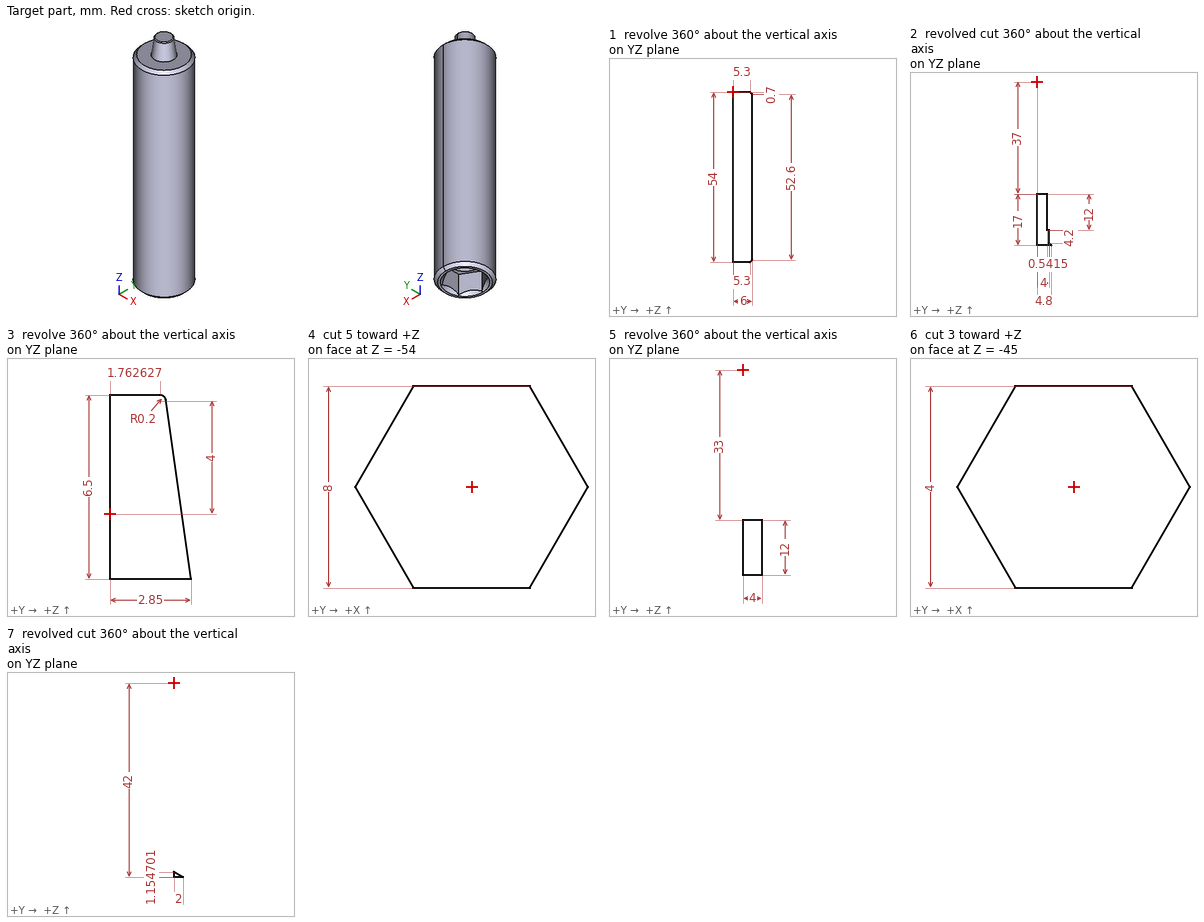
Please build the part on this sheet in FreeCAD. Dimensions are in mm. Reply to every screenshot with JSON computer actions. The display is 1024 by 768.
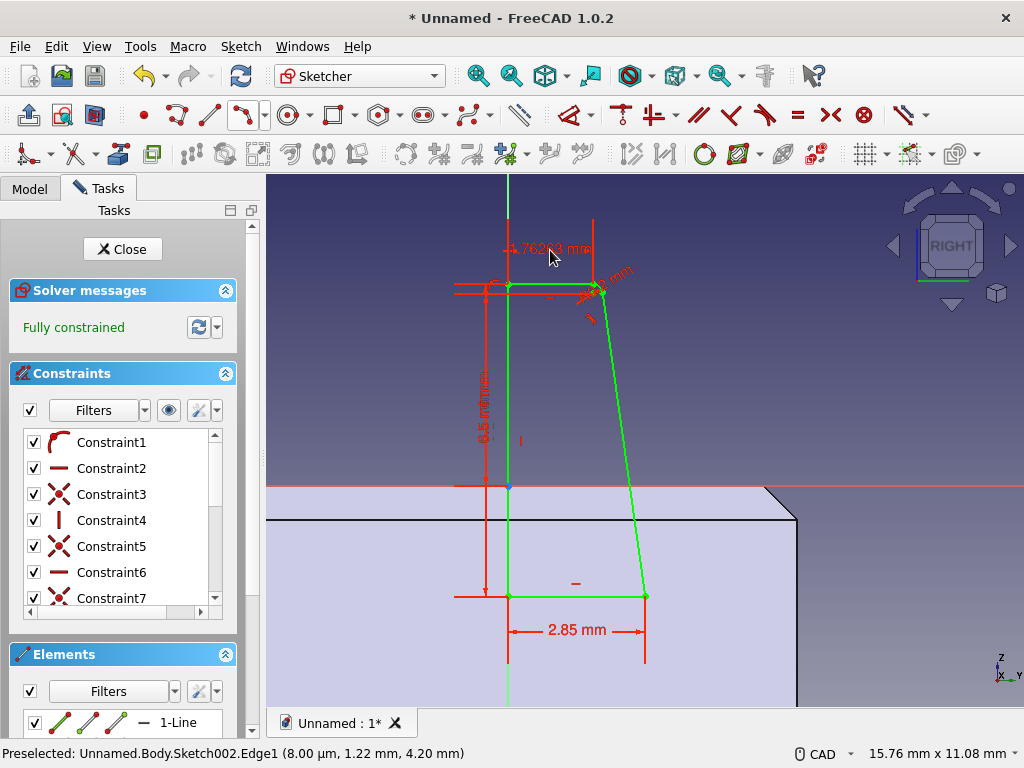
{"action": "left_click", "coordinate": [123, 249]}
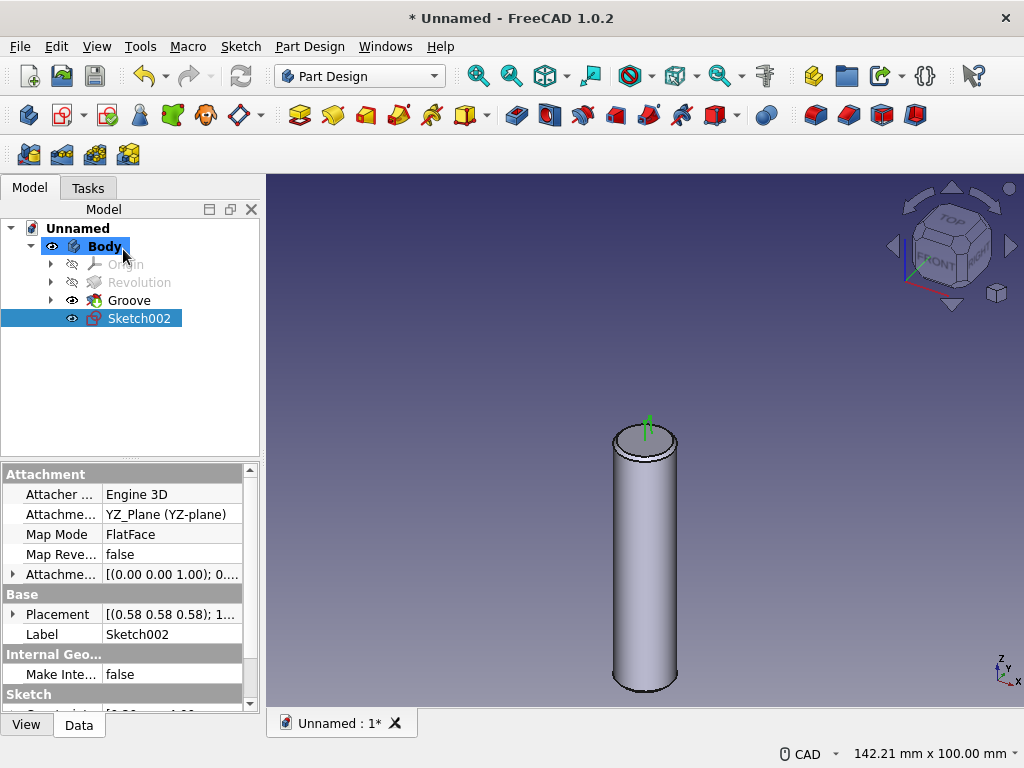
{"action": "left_click", "coordinate": [333, 116]}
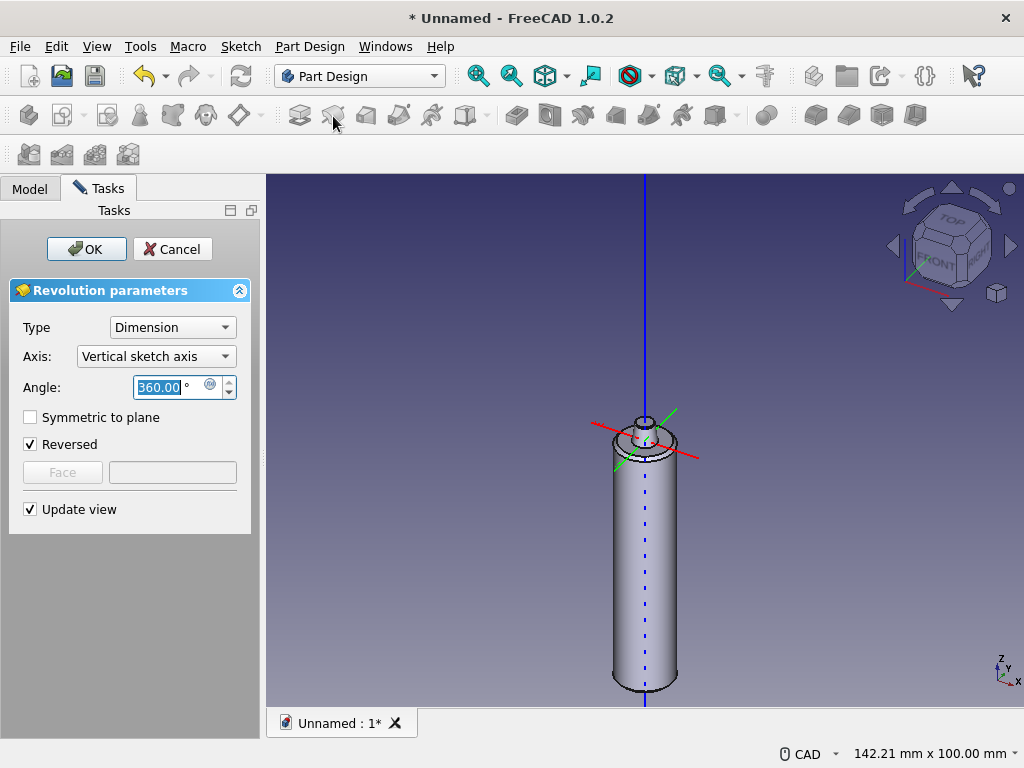
{"action": "left_click", "coordinate": [87, 249]}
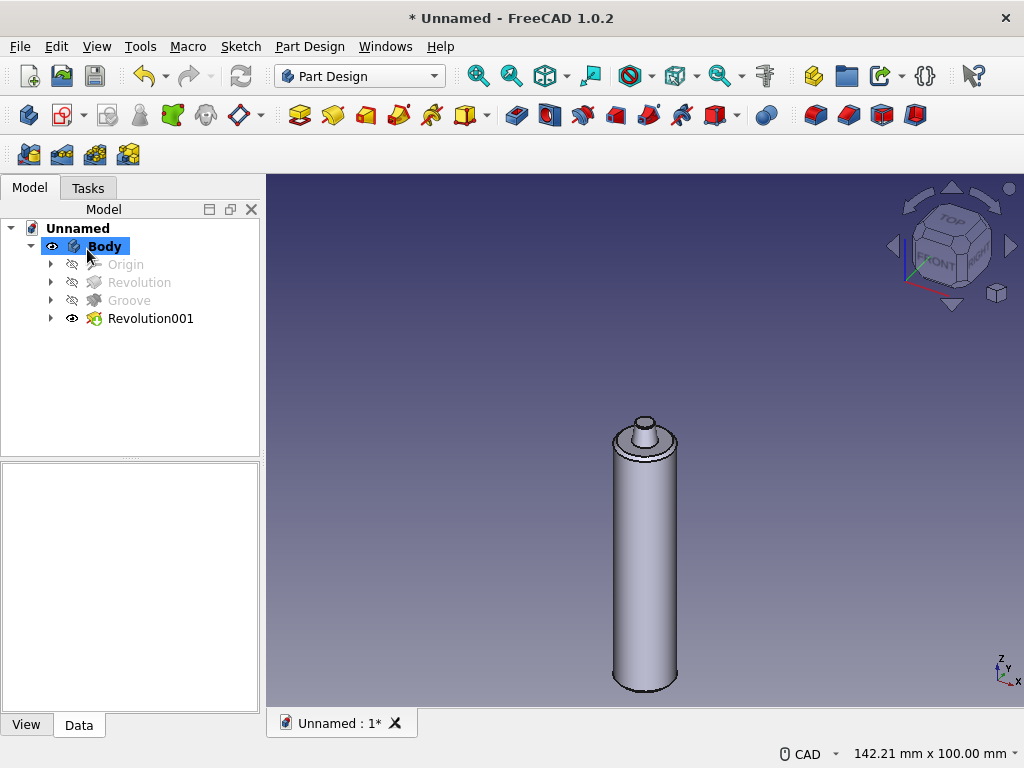
{"action": "key", "text": "5"}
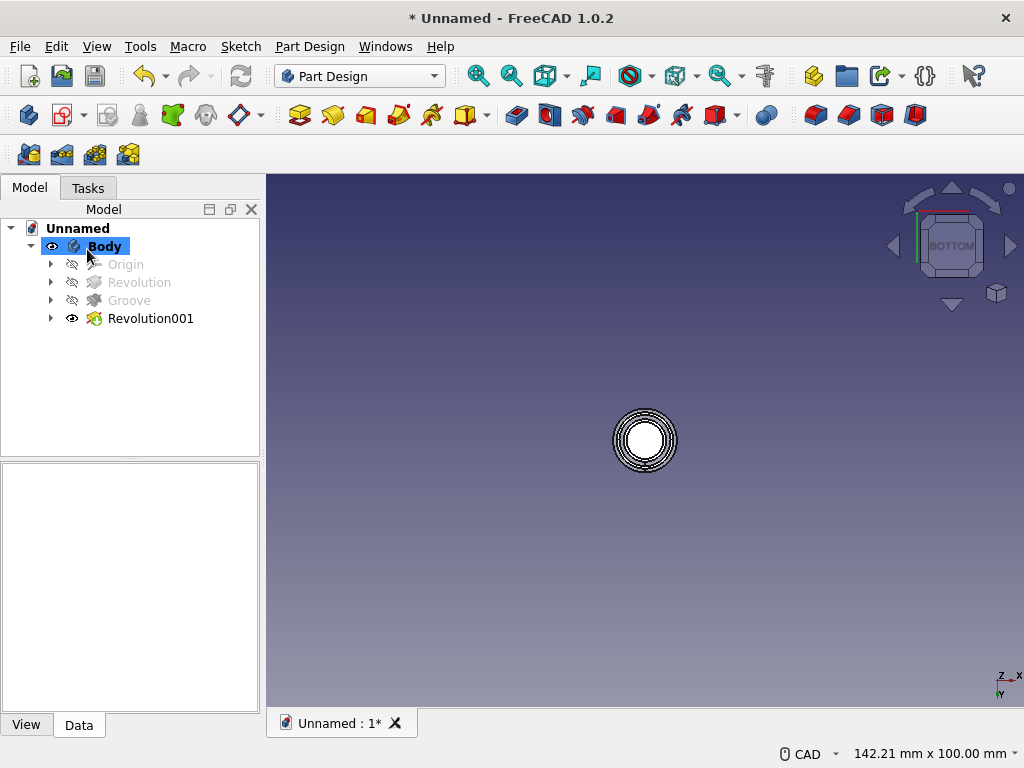
{"action": "left_click", "coordinate": [479, 76]}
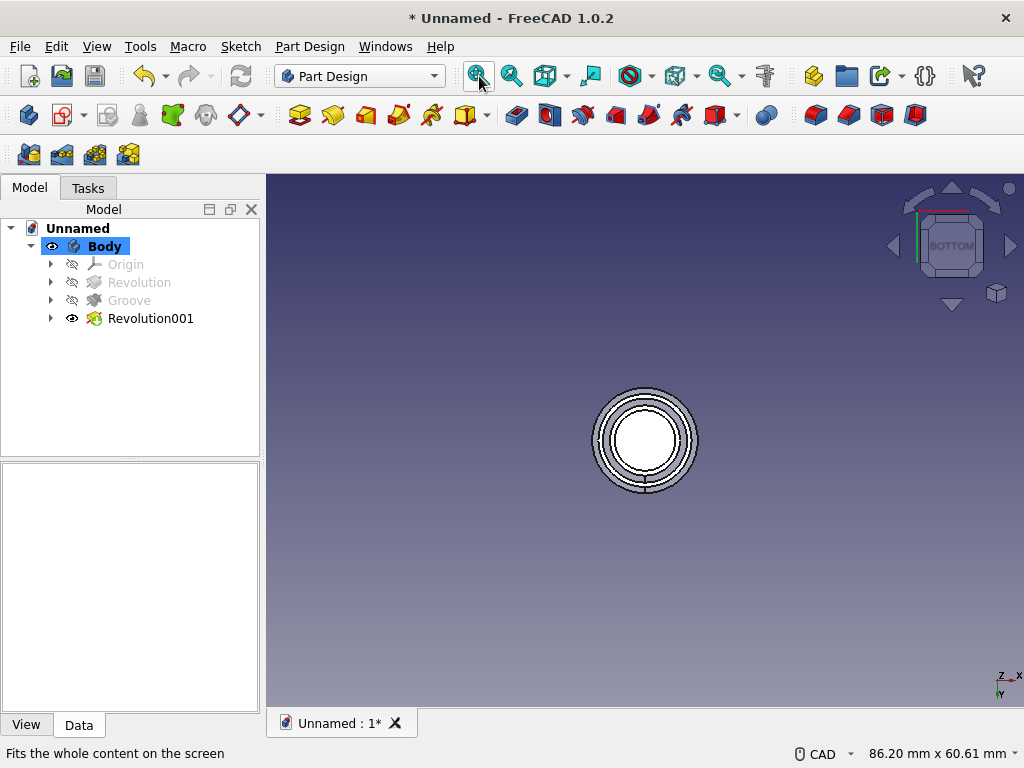
{"action": "scroll", "coordinate": [618, 403], "scroll_direction": "up", "scroll_amount": 11}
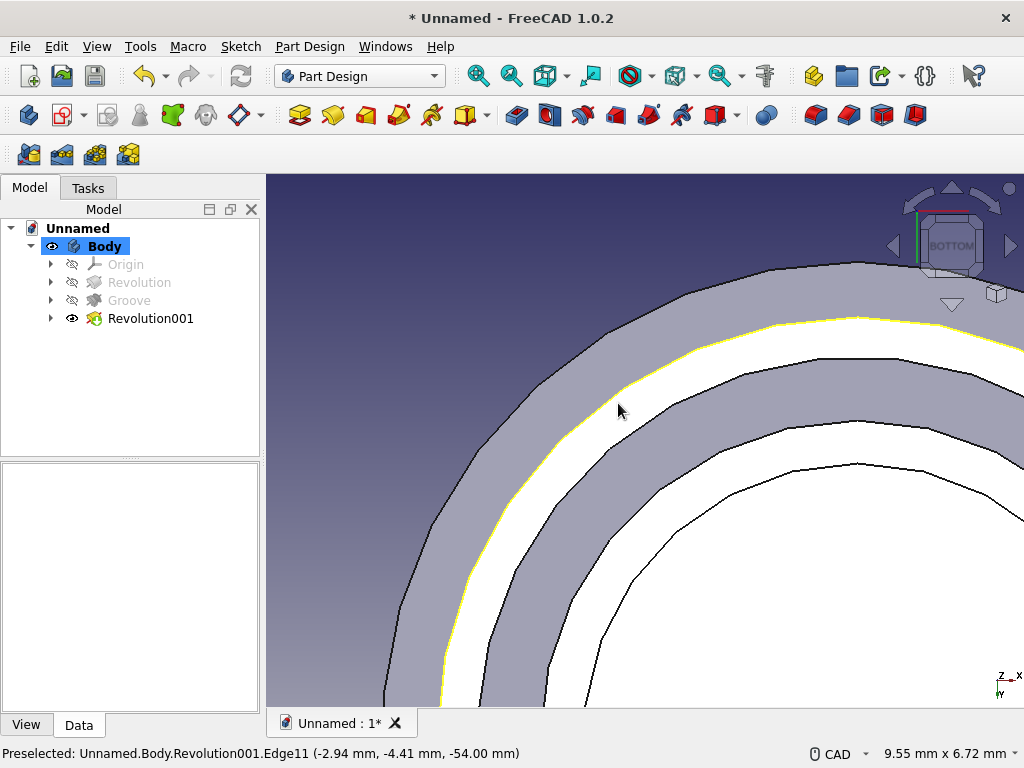
{"action": "left_click", "coordinate": [618, 408]}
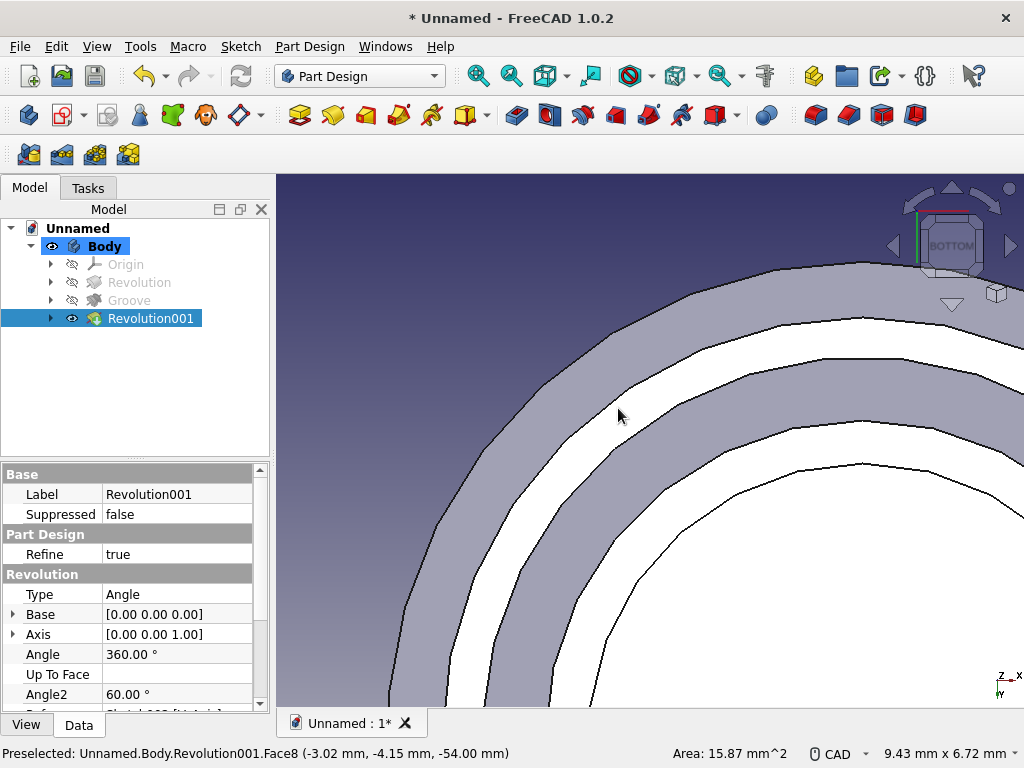
{"action": "left_click", "coordinate": [62, 116]}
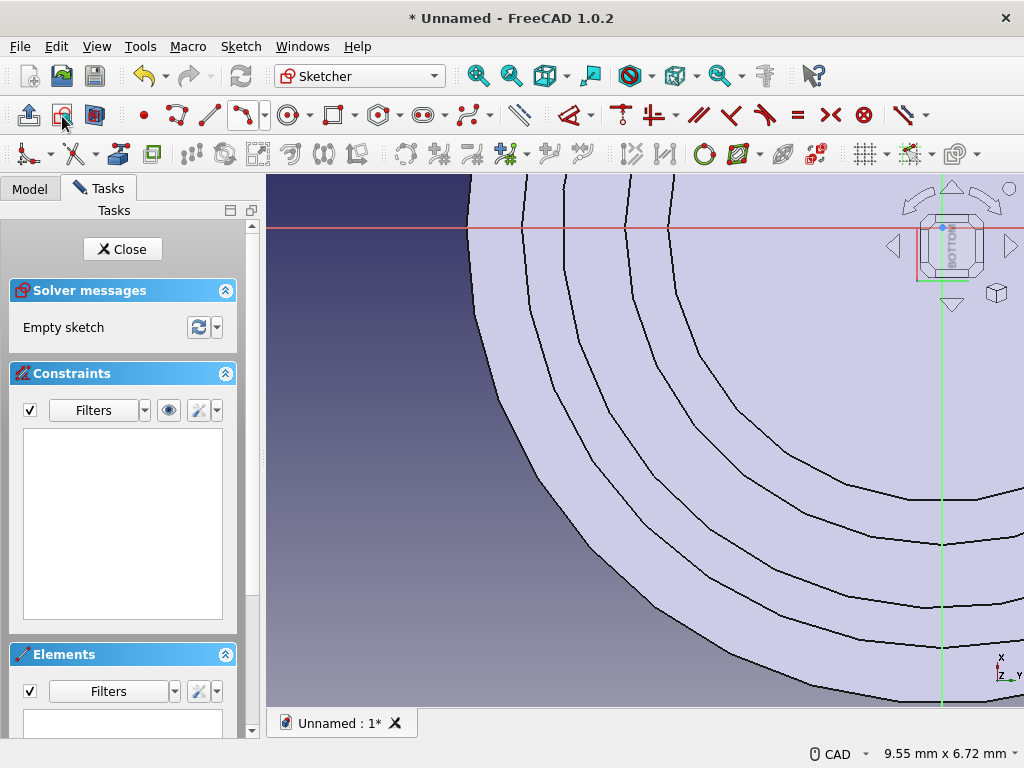
{"action": "scroll", "coordinate": [294, 614], "scroll_direction": "down", "scroll_amount": 4}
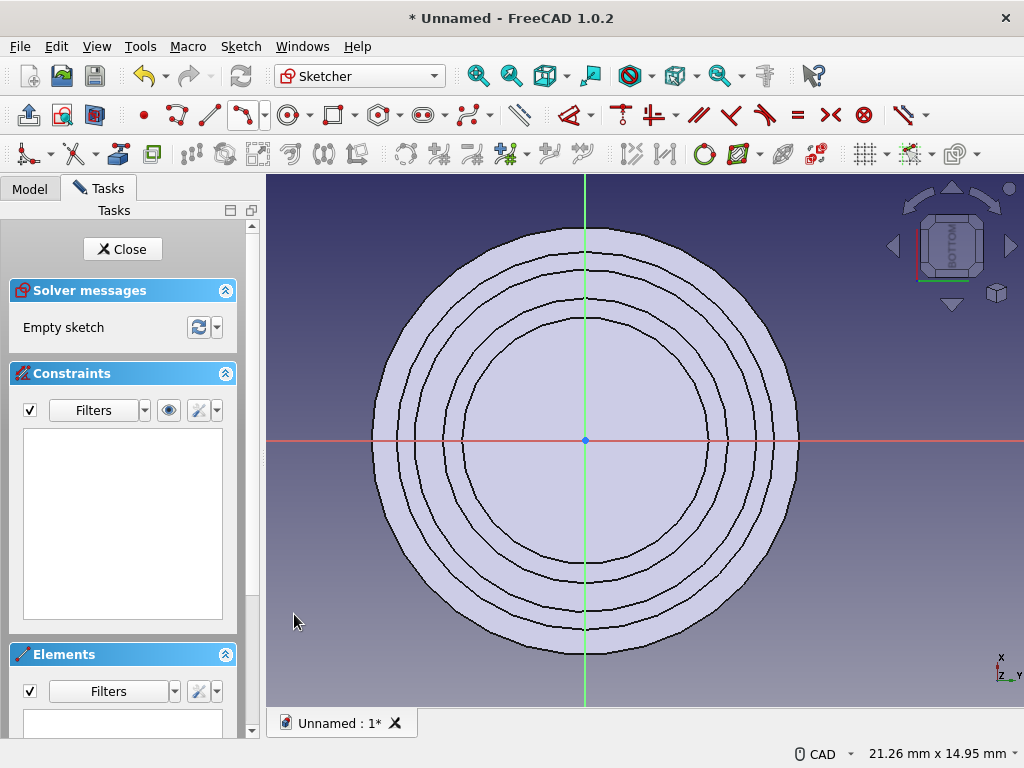
{"action": "left_click", "coordinate": [378, 116]}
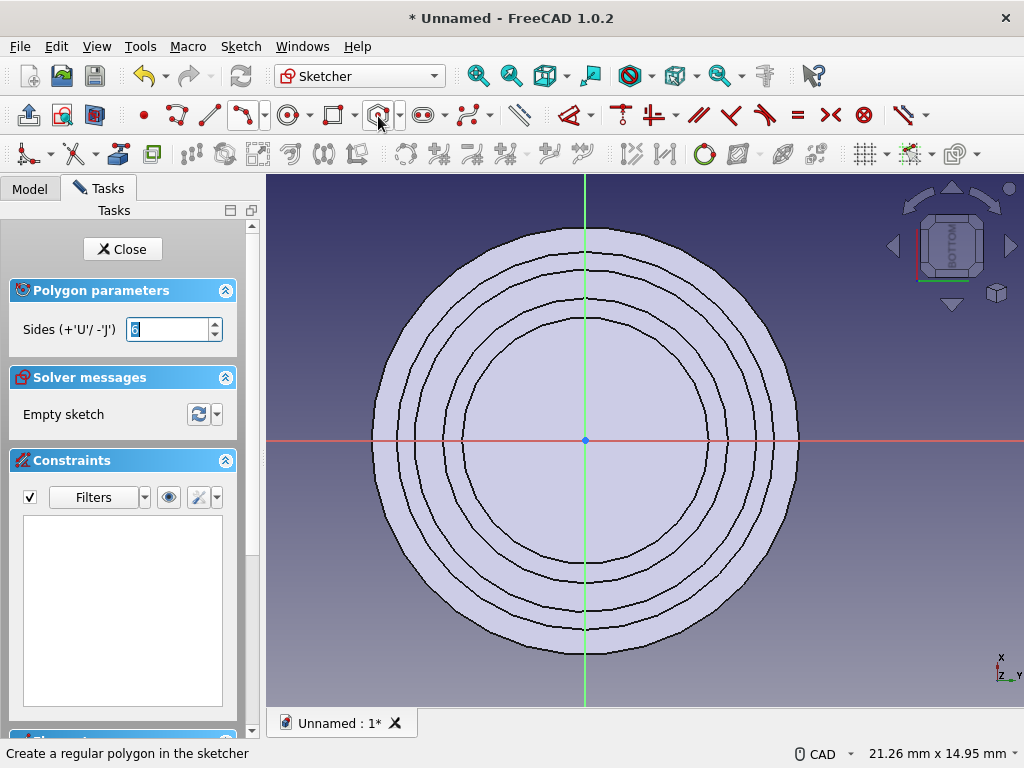
{"action": "left_click", "coordinate": [585, 441]}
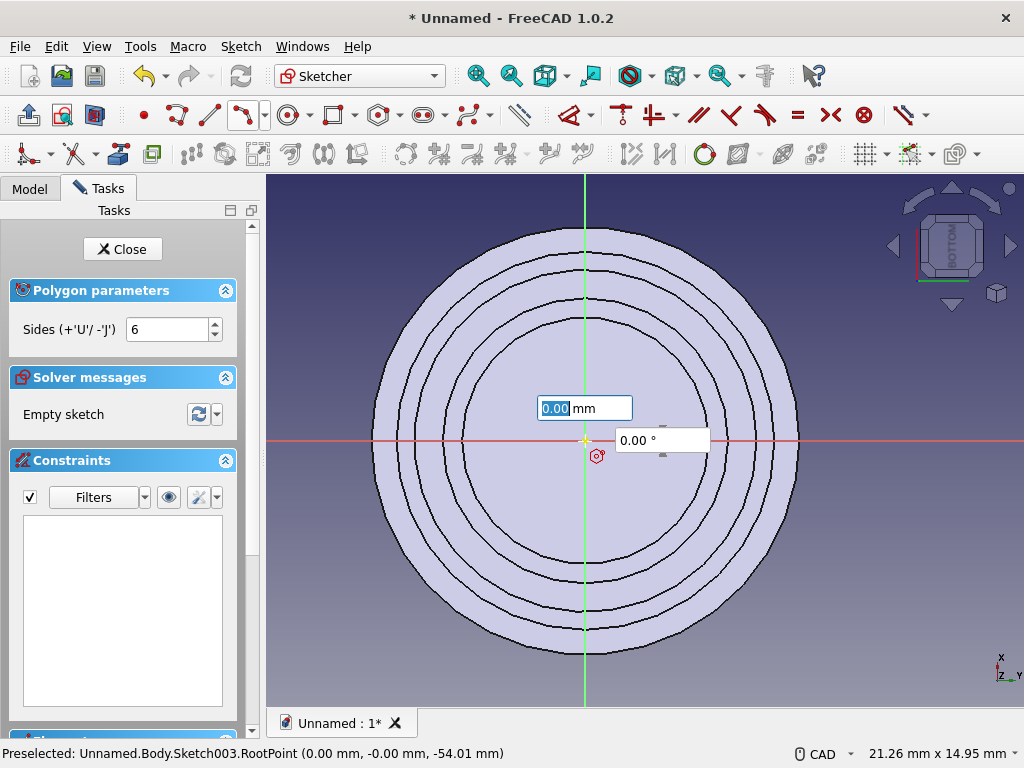
{"action": "left_click", "coordinate": [421, 441]}
{"action": "right_click", "coordinate": [421, 441]}